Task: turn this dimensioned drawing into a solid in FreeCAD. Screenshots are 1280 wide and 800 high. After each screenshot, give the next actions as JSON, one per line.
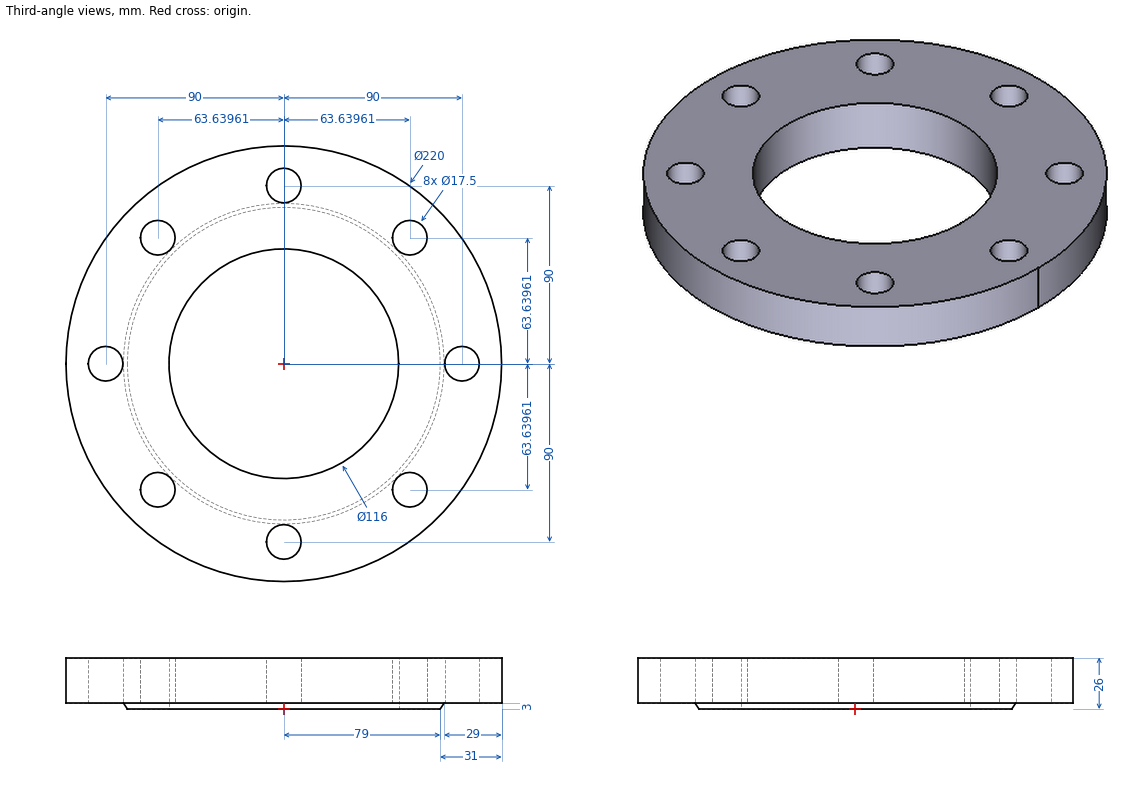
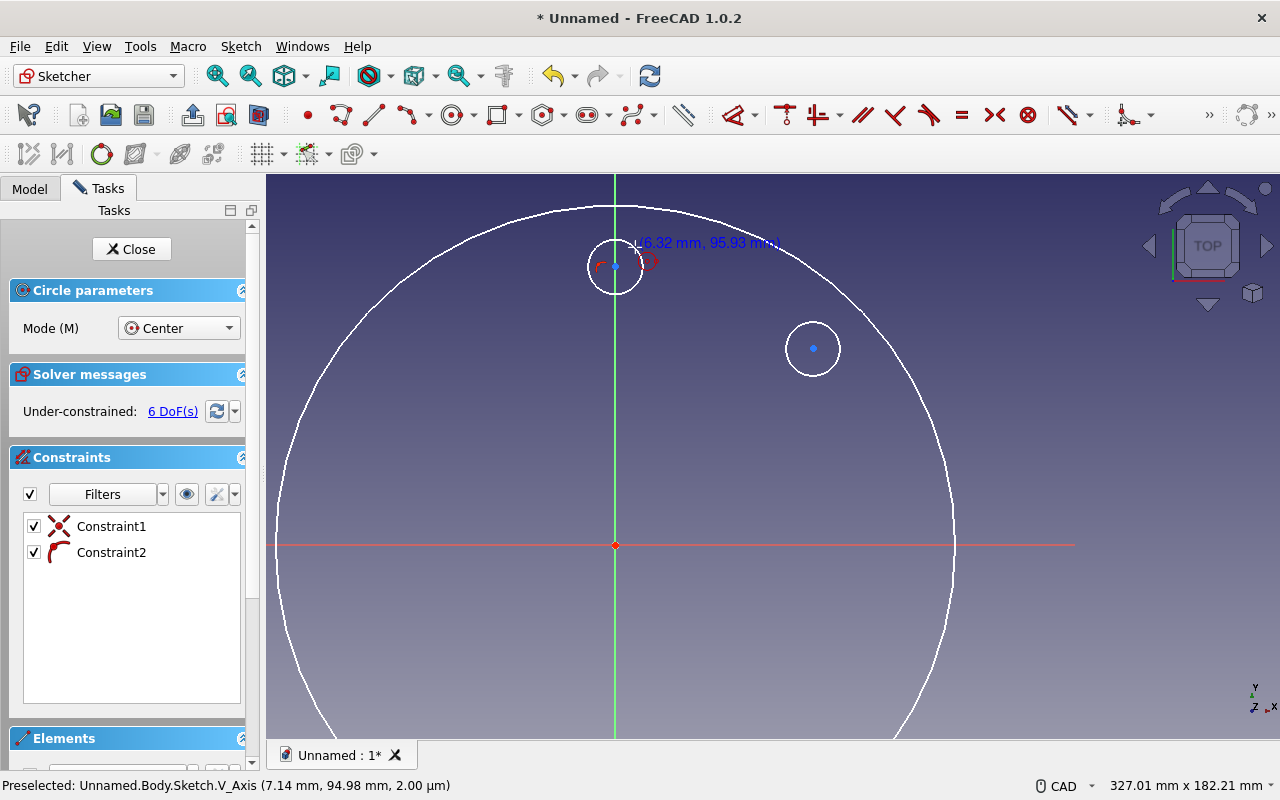
{"action": "left_click", "coordinate": [418, 348]}
{"action": "left_click", "coordinate": [437, 329]}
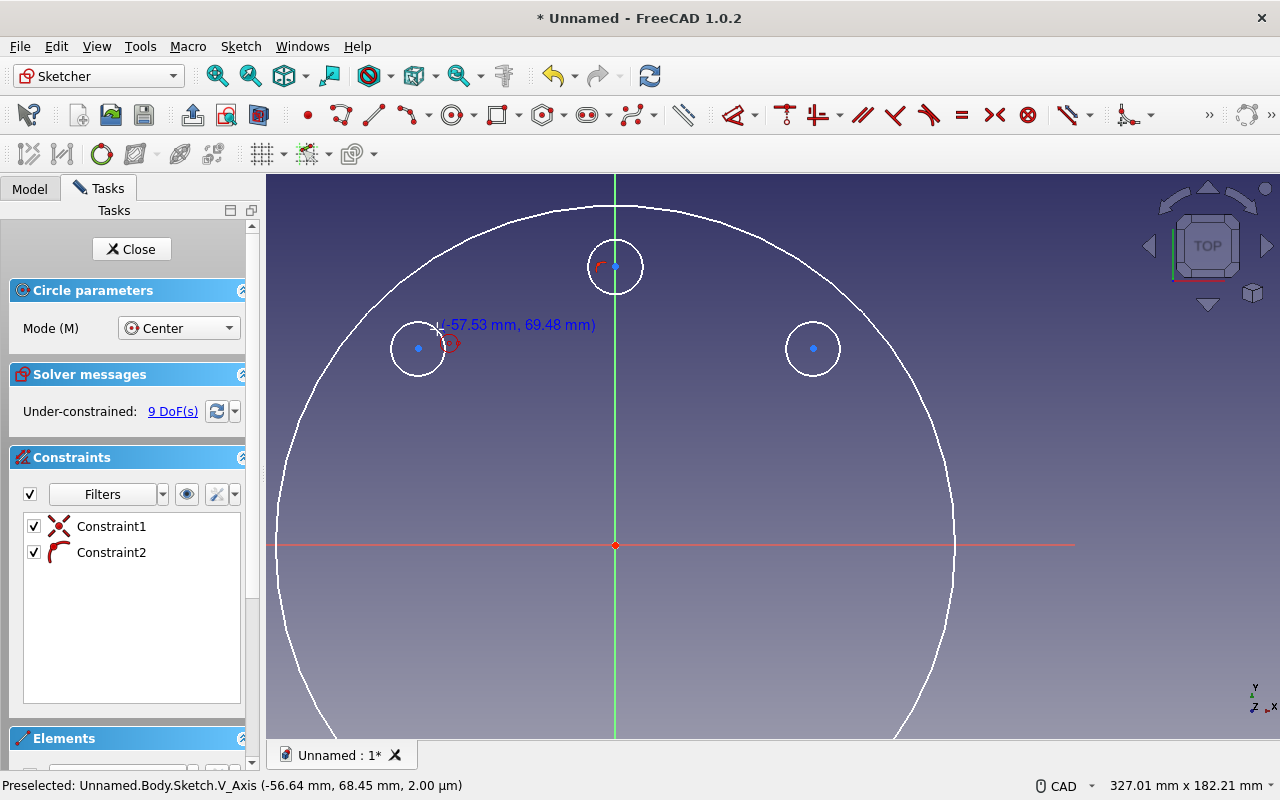
{"action": "left_click", "coordinate": [894, 545]}
{"action": "left_click", "coordinate": [914, 526]}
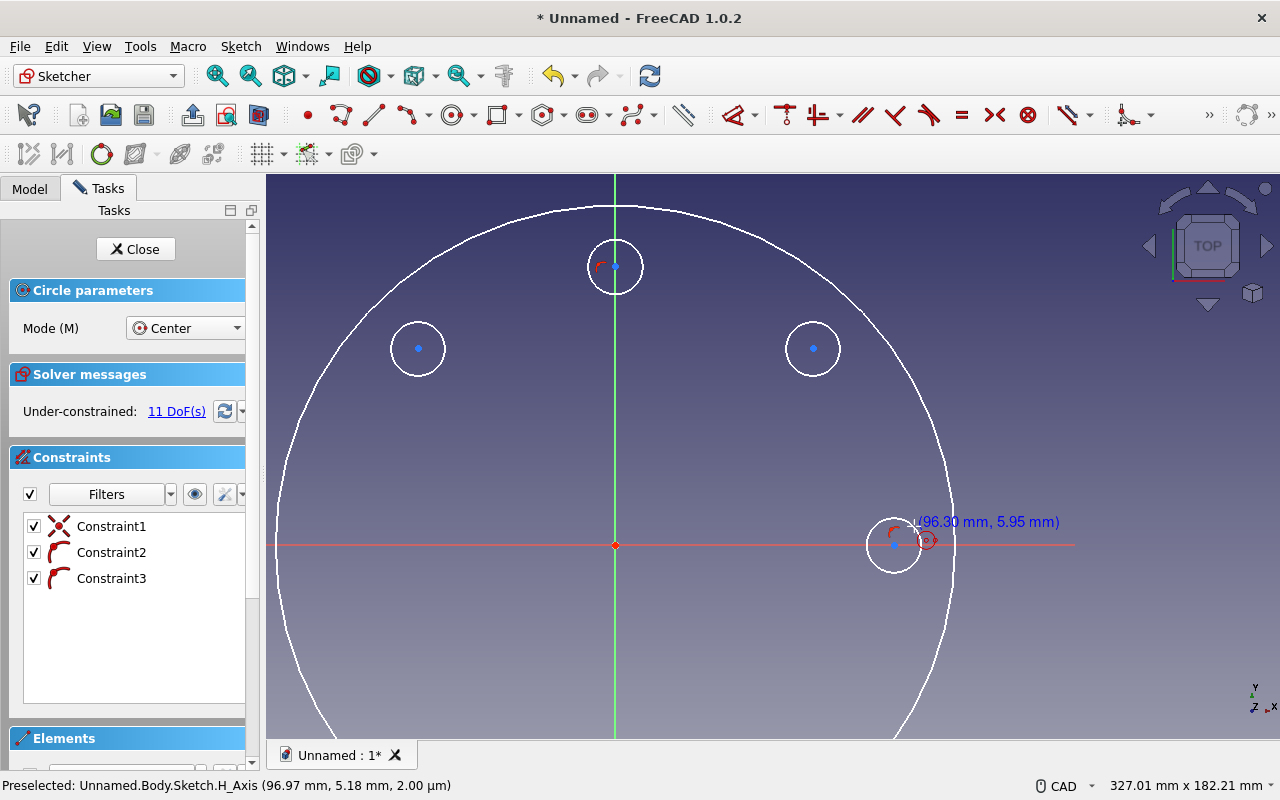
{"action": "scroll", "coordinate": [813, 348], "scroll_direction": "down", "scroll_amount": 3}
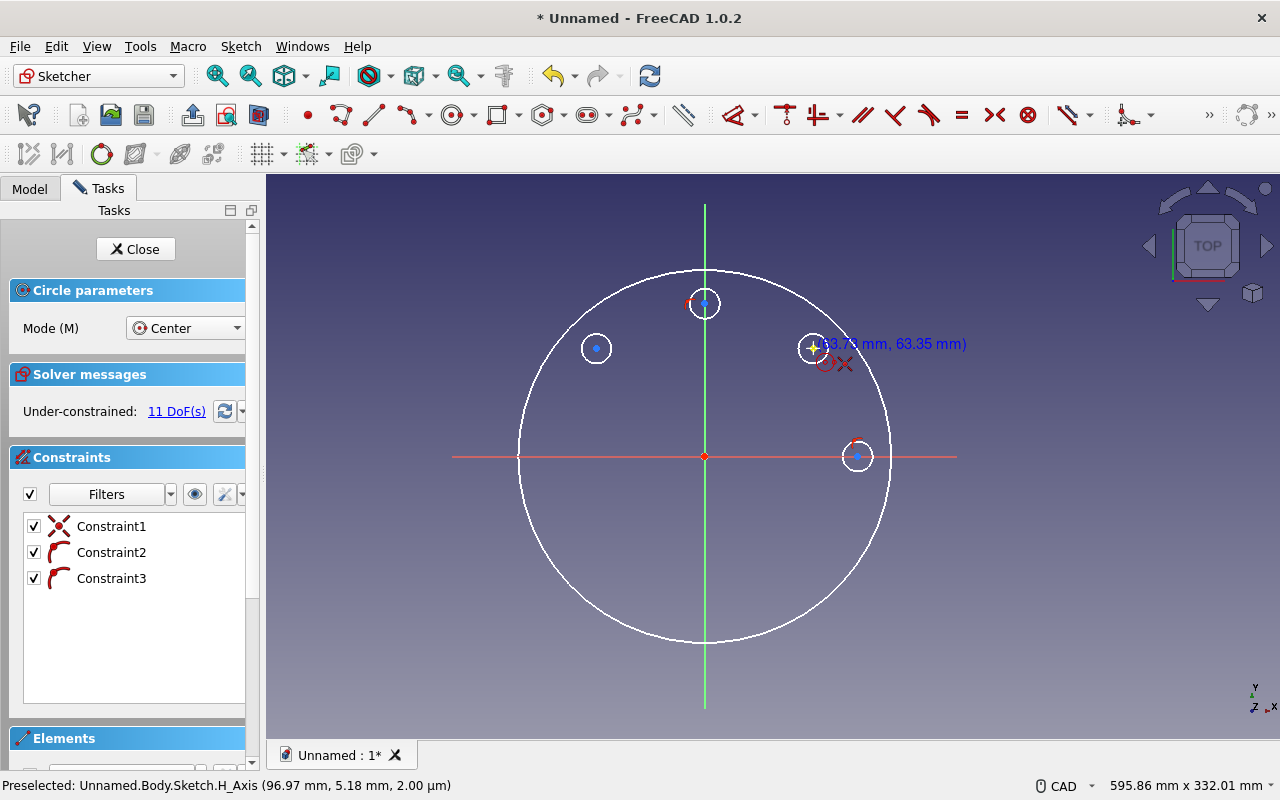
{"action": "scroll", "coordinate": [813, 565], "scroll_direction": "up", "scroll_amount": 3}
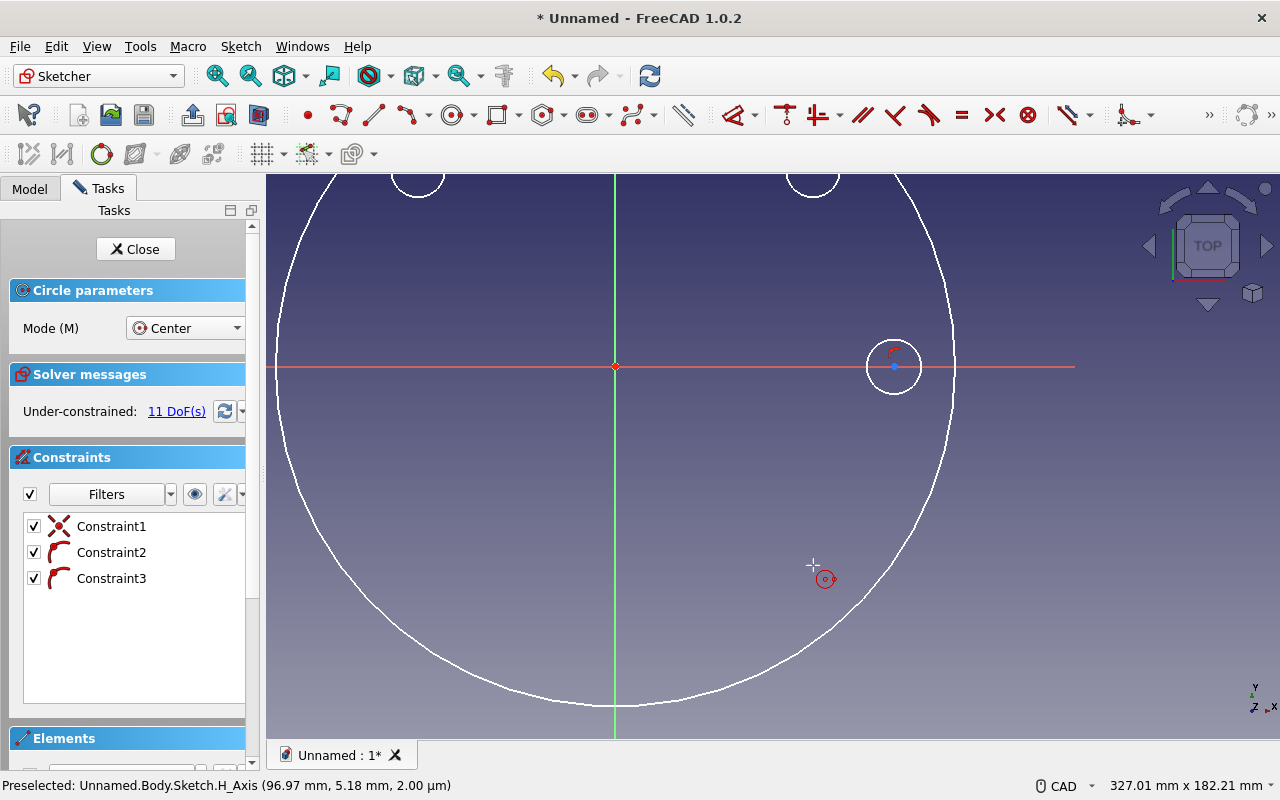
{"action": "left_click", "coordinate": [813, 564]}
{"action": "left_click", "coordinate": [832, 545]}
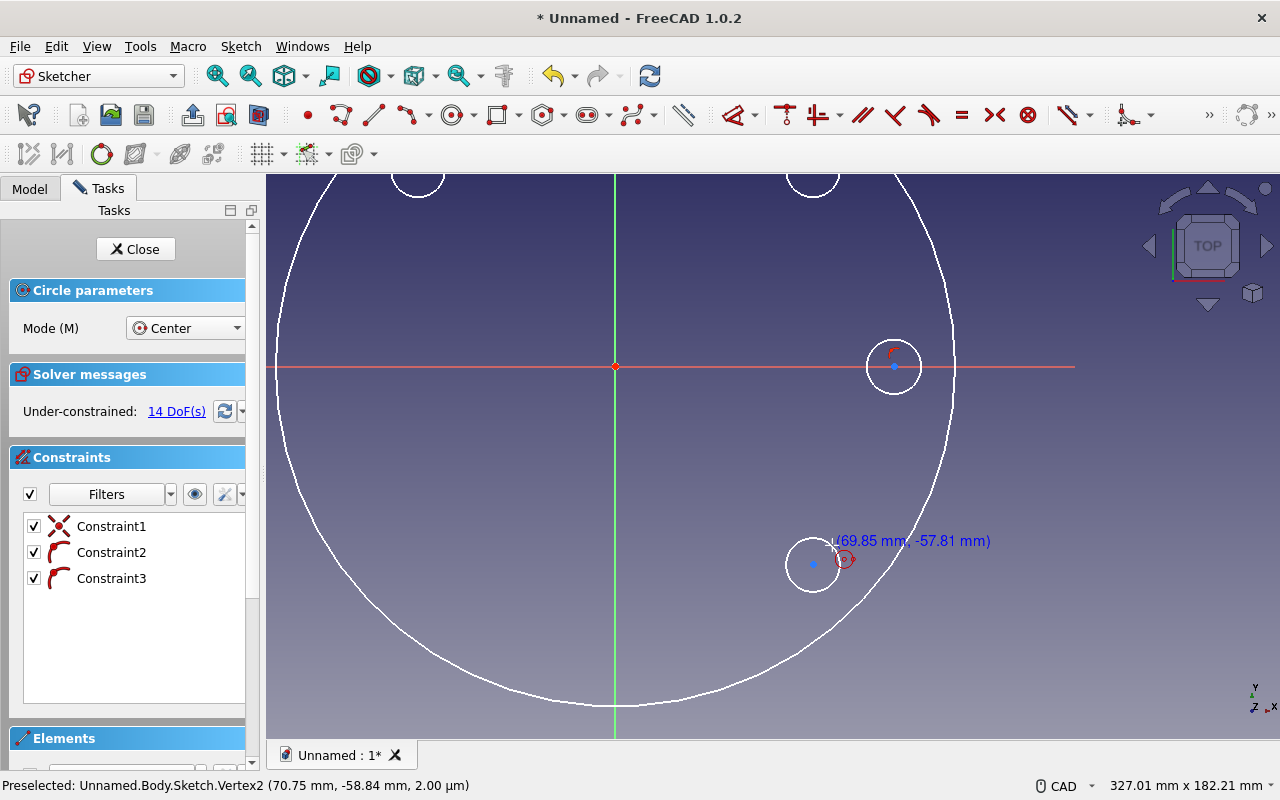
{"action": "left_click", "coordinate": [336, 367]}
{"action": "left_click", "coordinate": [356, 348]}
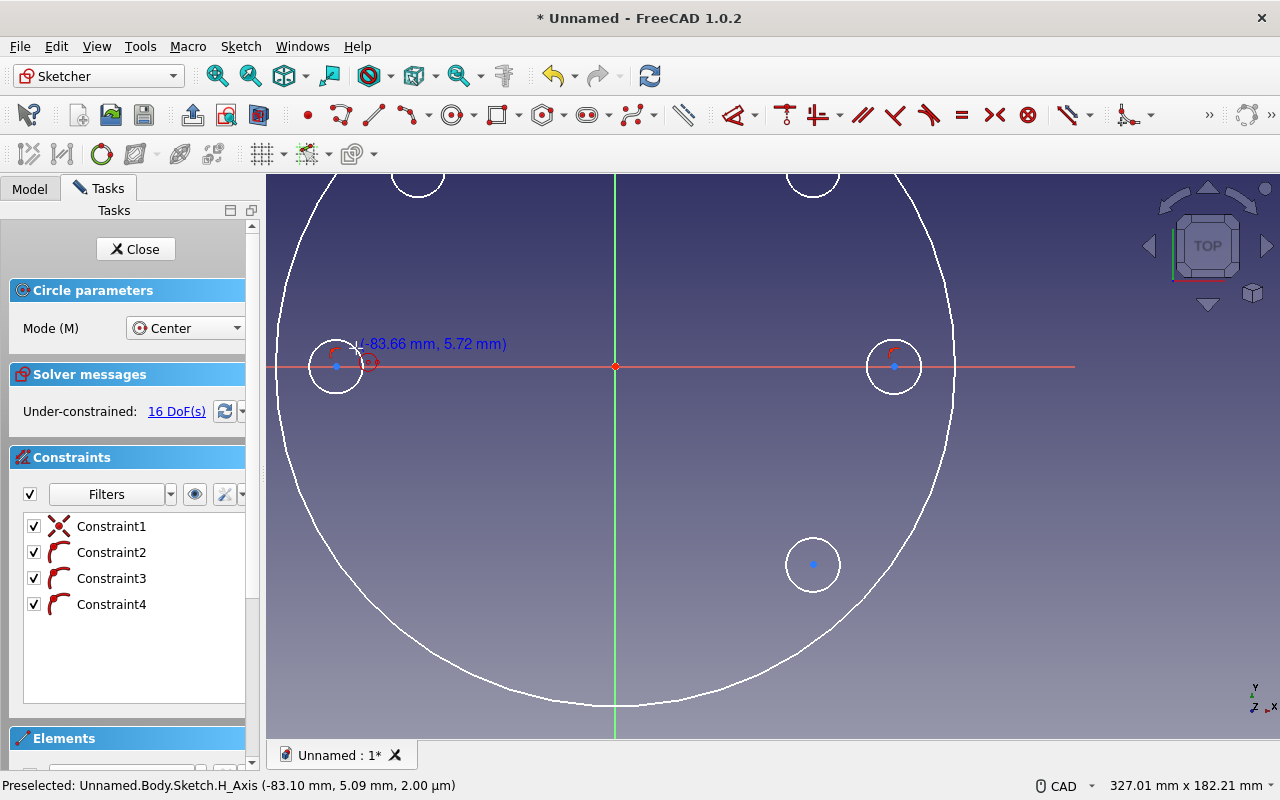
{"action": "left_click", "coordinate": [615, 646]}
{"action": "left_click", "coordinate": [635, 627]}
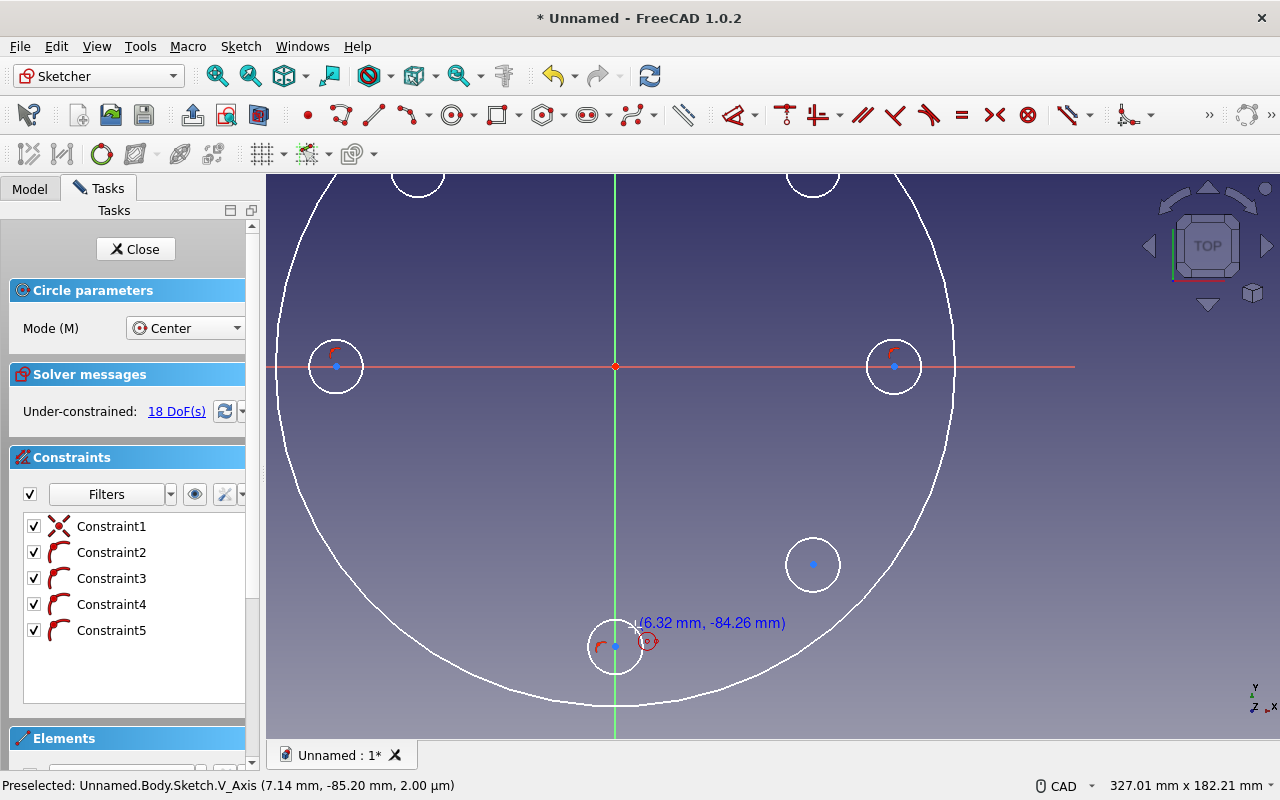
{"action": "left_click", "coordinate": [418, 564]}
{"action": "left_click", "coordinate": [437, 545]}
{"action": "key", "text": "Escape"}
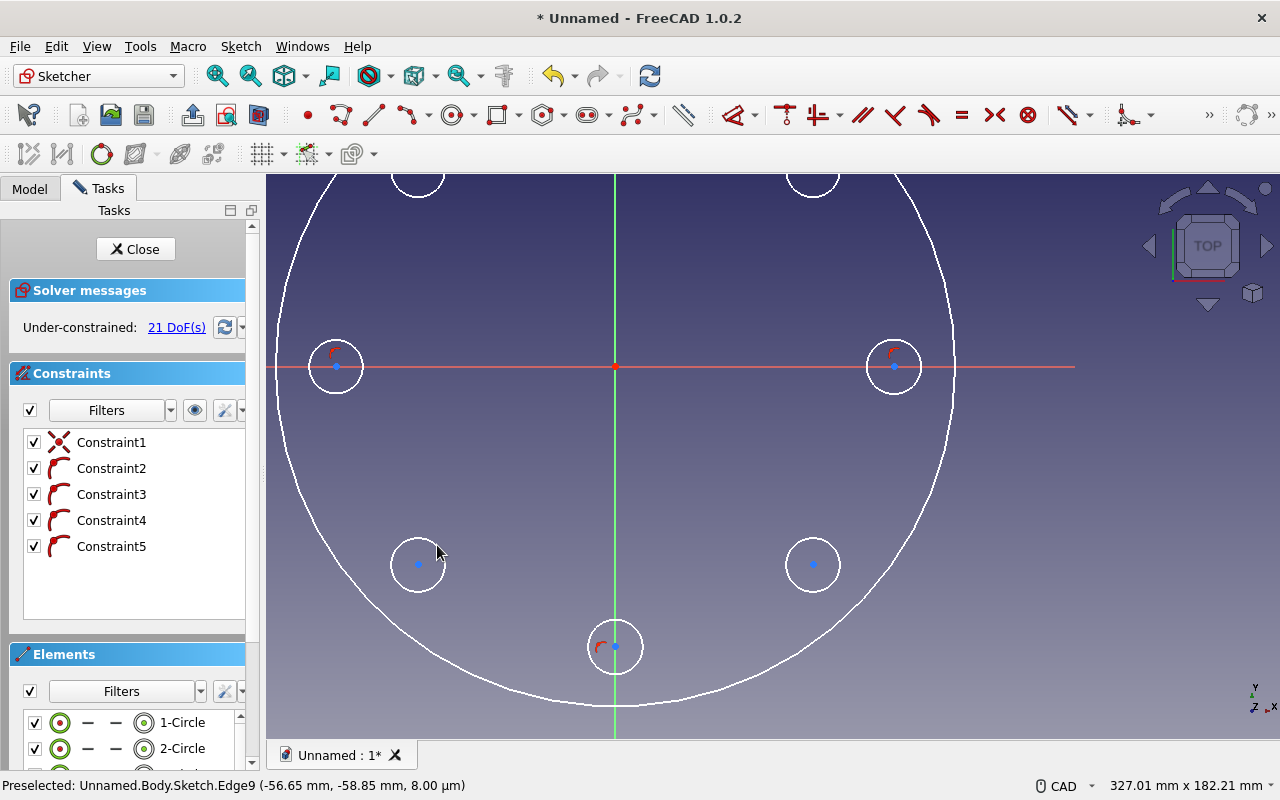
{"action": "scroll", "coordinate": [813, 566], "scroll_direction": "down", "scroll_amount": 3}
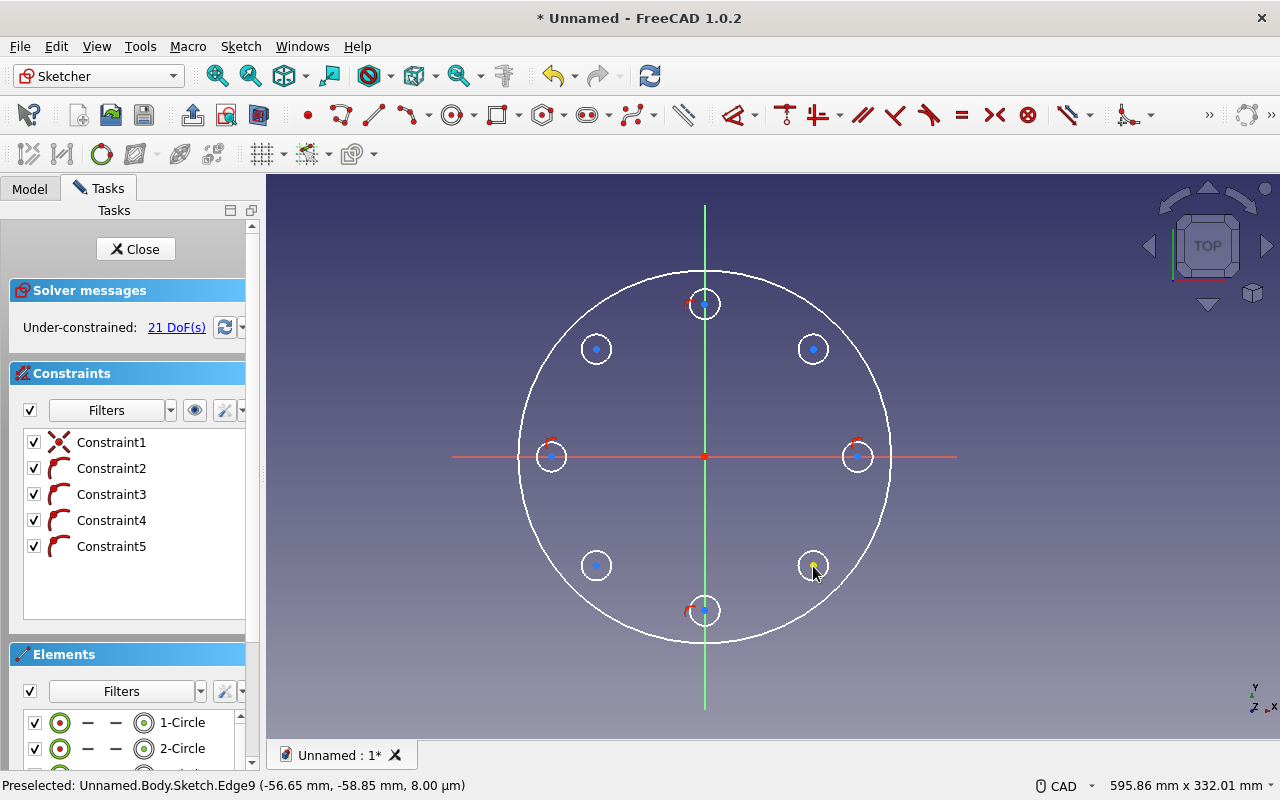
{"action": "left_click", "coordinate": [824, 339]}